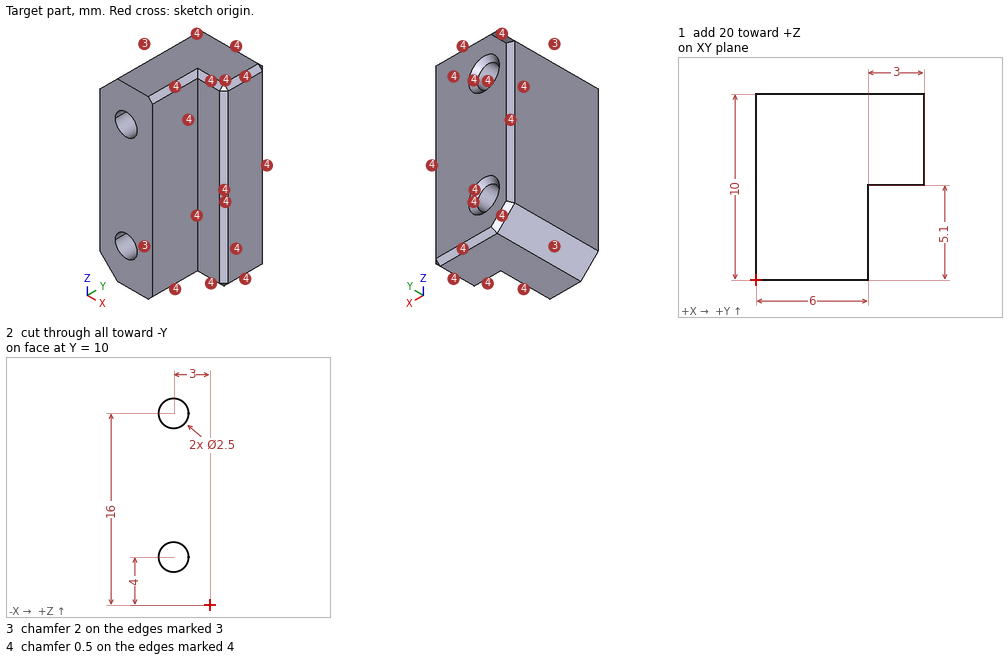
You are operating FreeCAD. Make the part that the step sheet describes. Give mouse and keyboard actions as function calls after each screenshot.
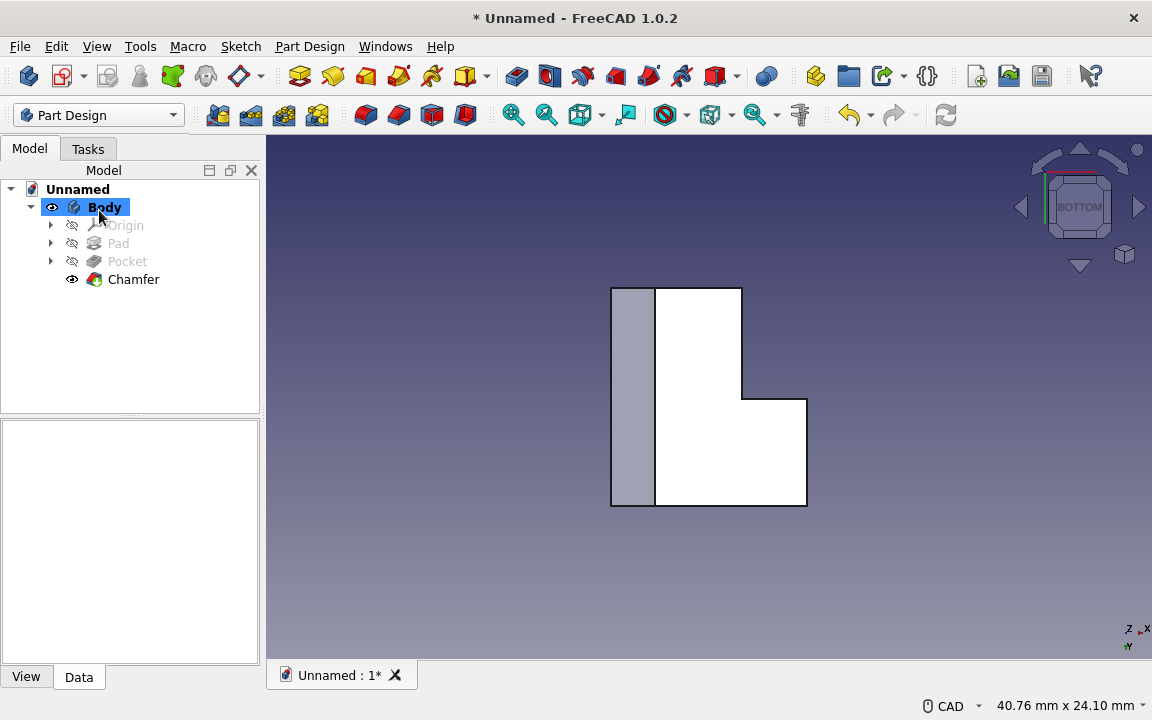
click(514, 116)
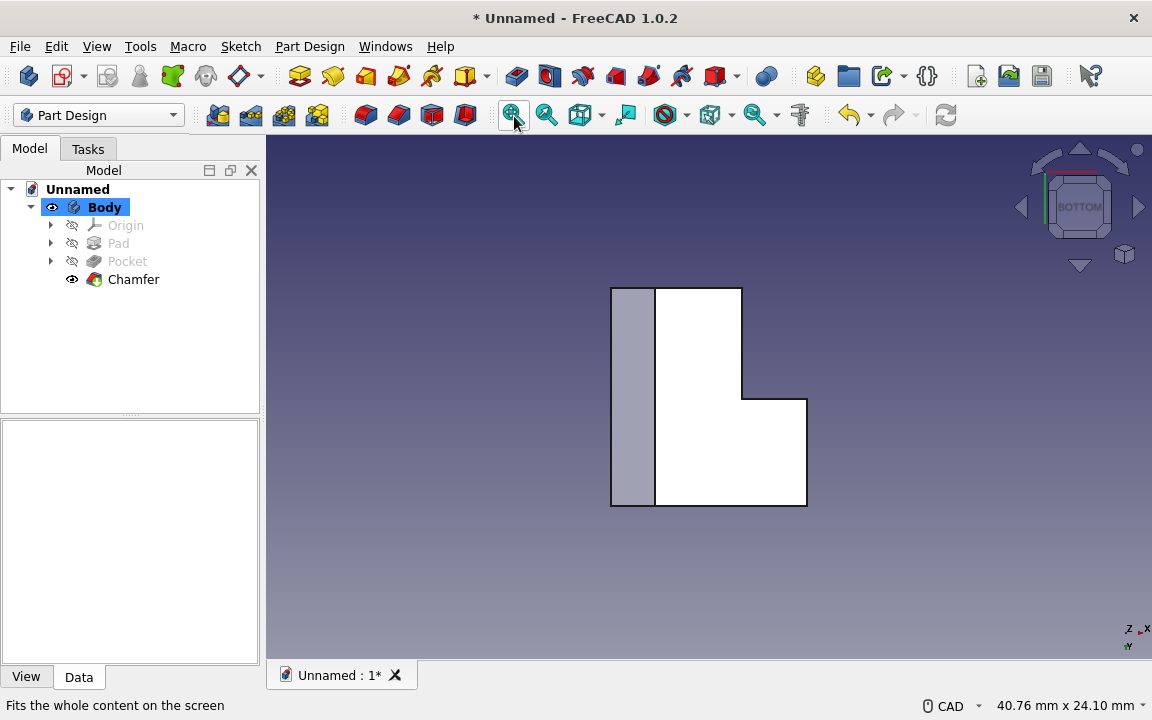
click(774, 398)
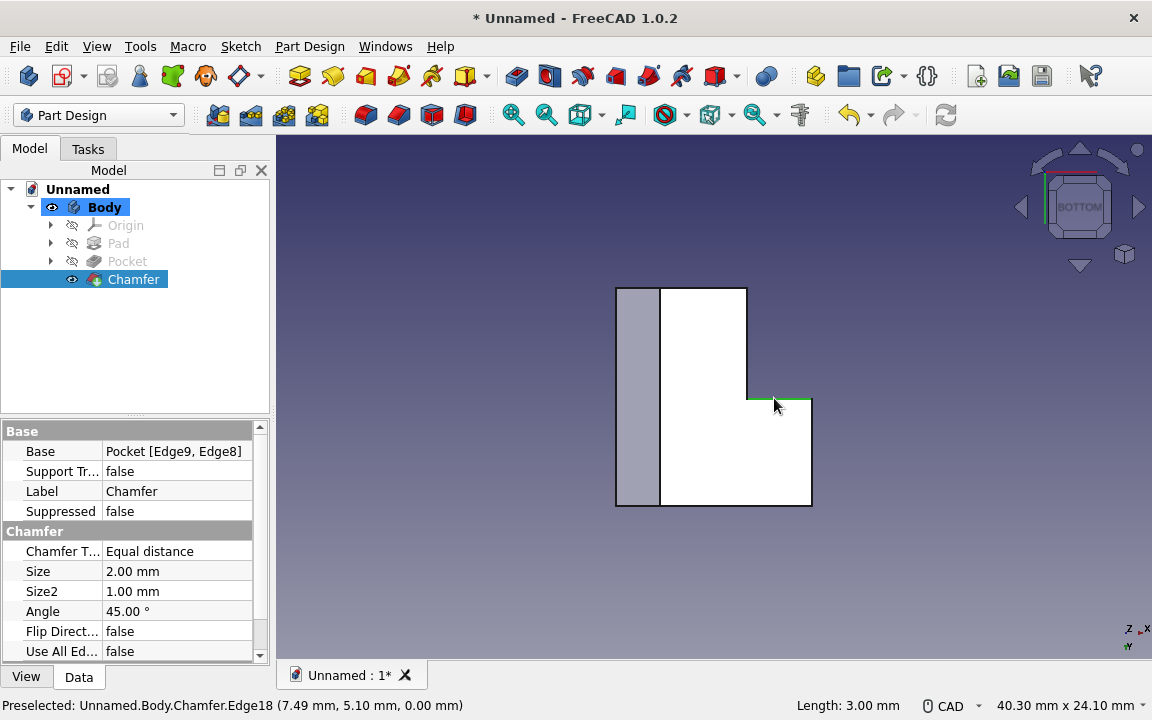
key(0)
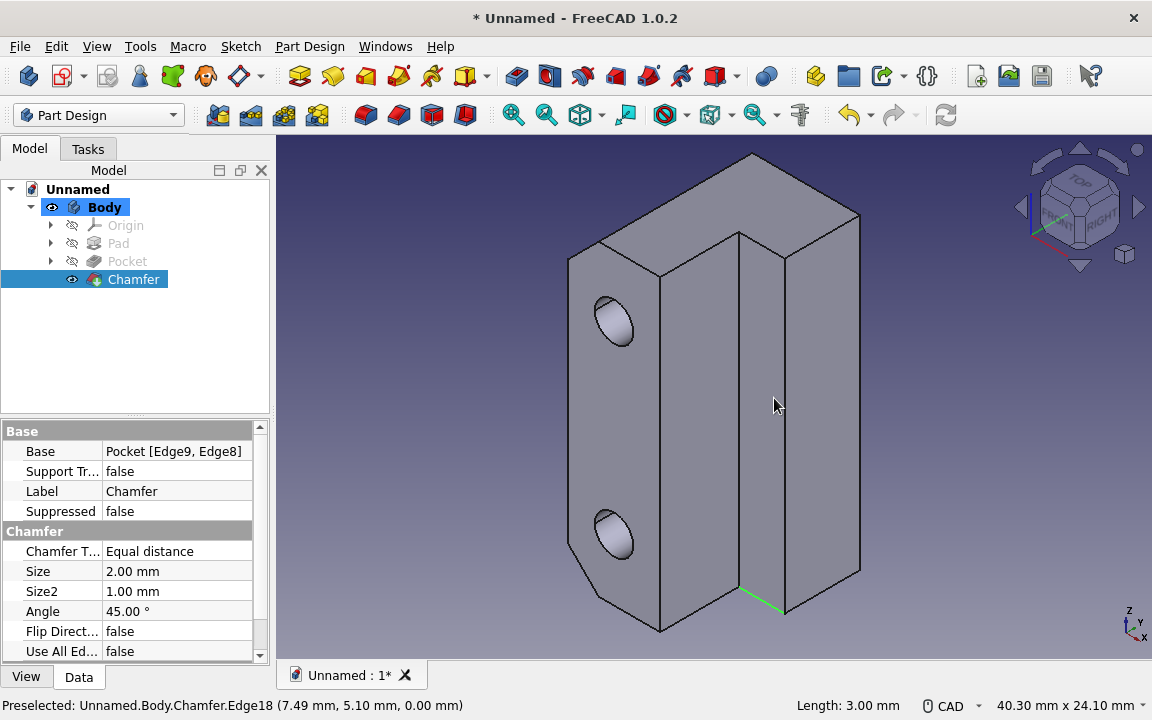
click(514, 116)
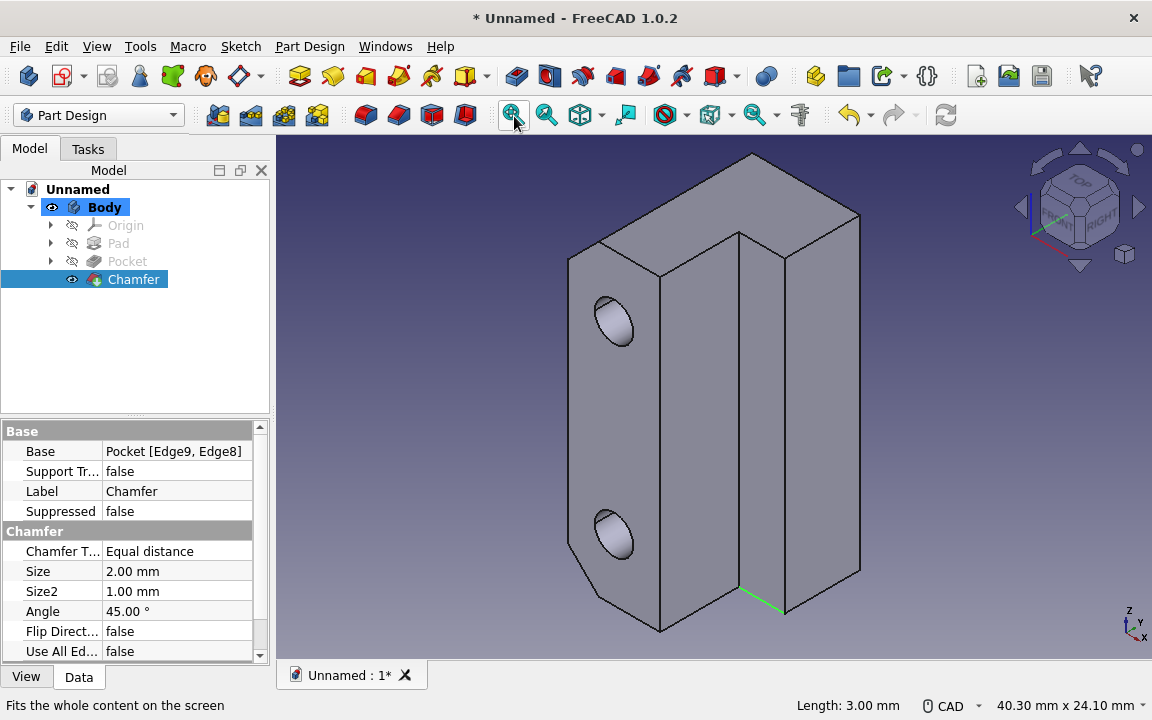
click(822, 312, ctrl)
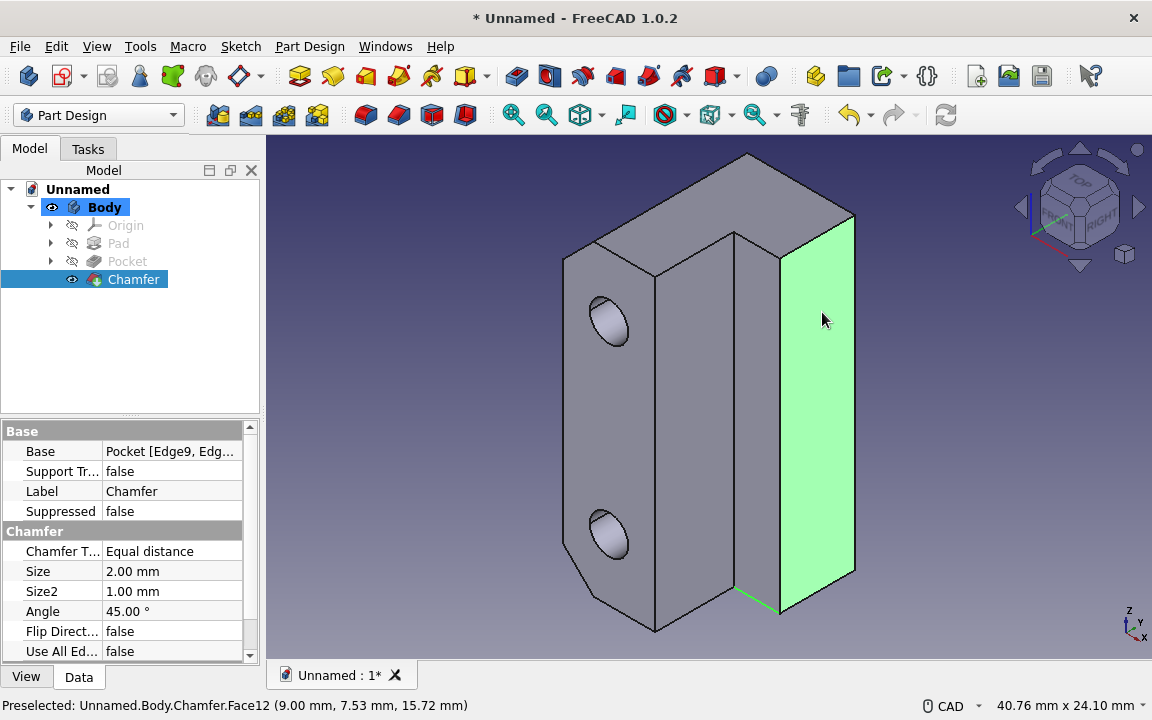
click(694, 254, ctrl)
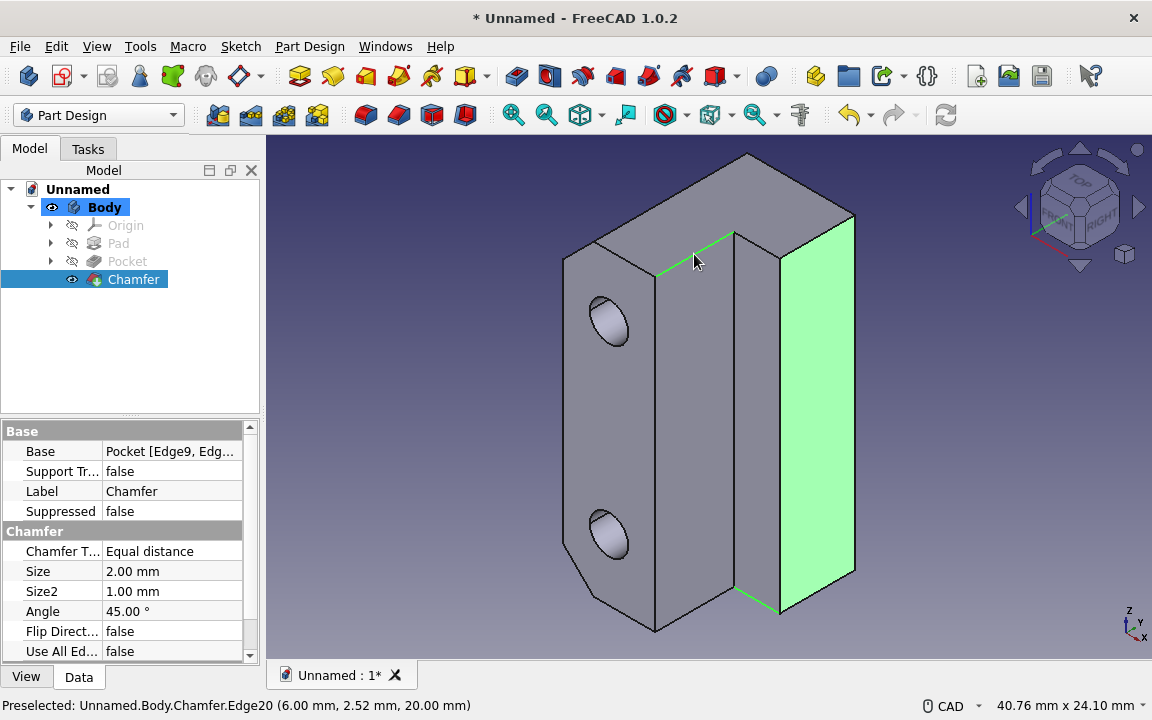
click(757, 244, ctrl)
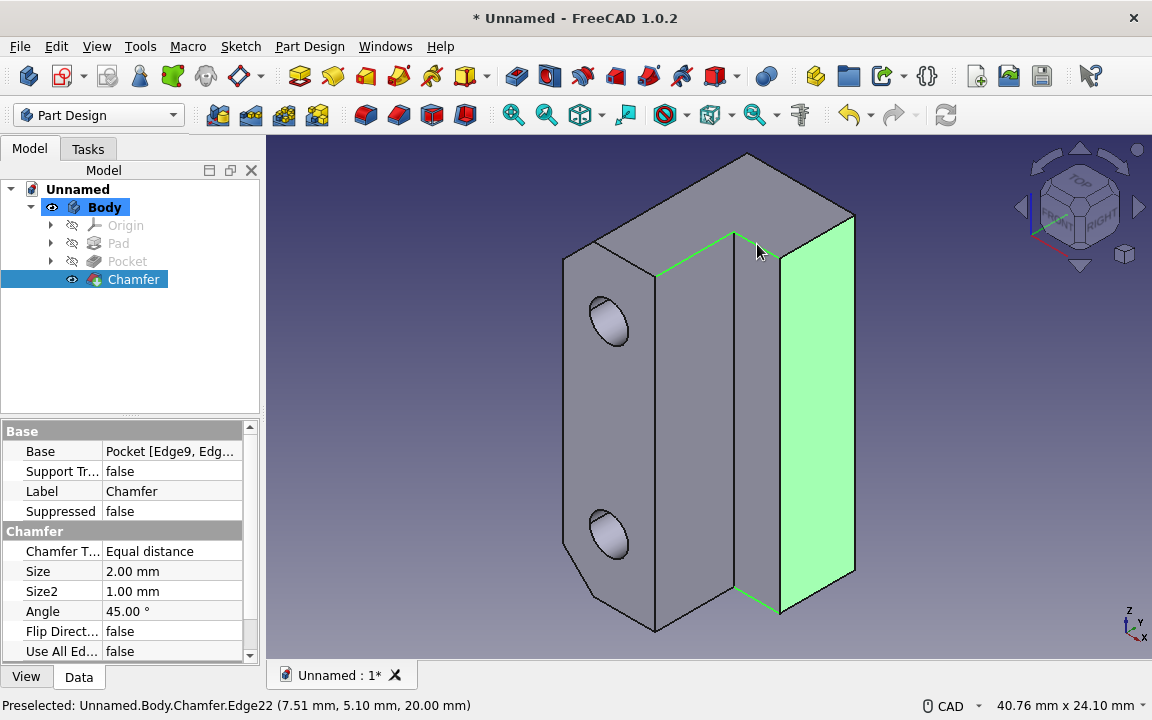
key(2)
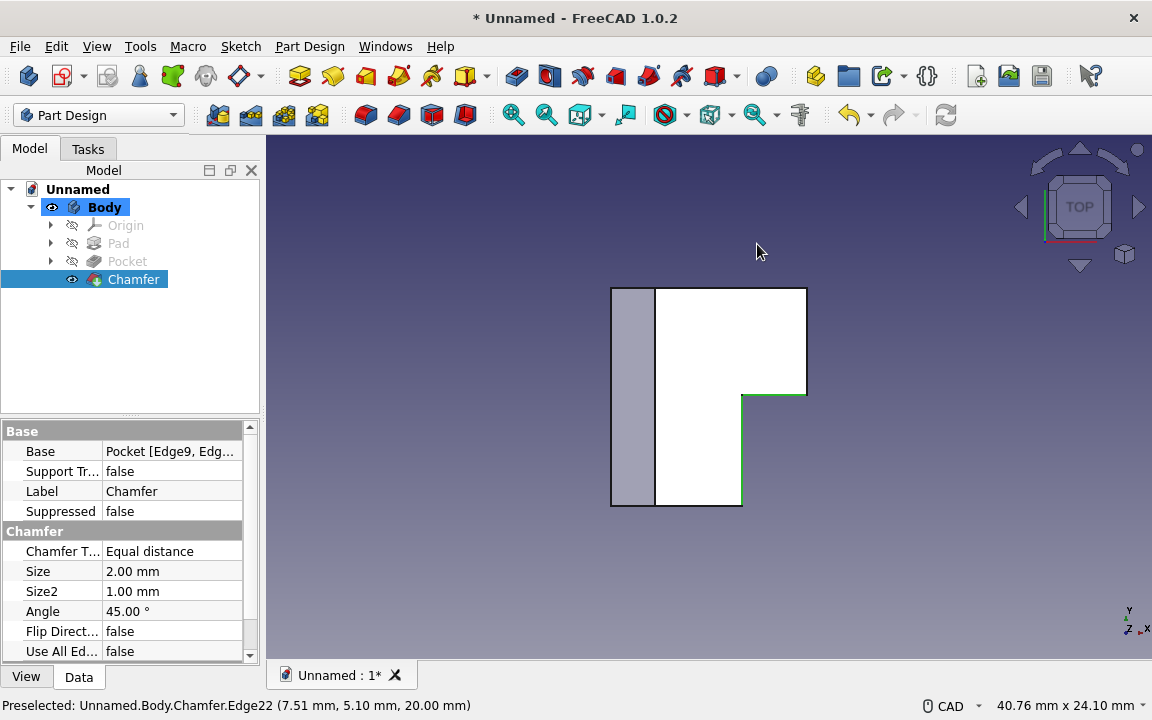
click(514, 116)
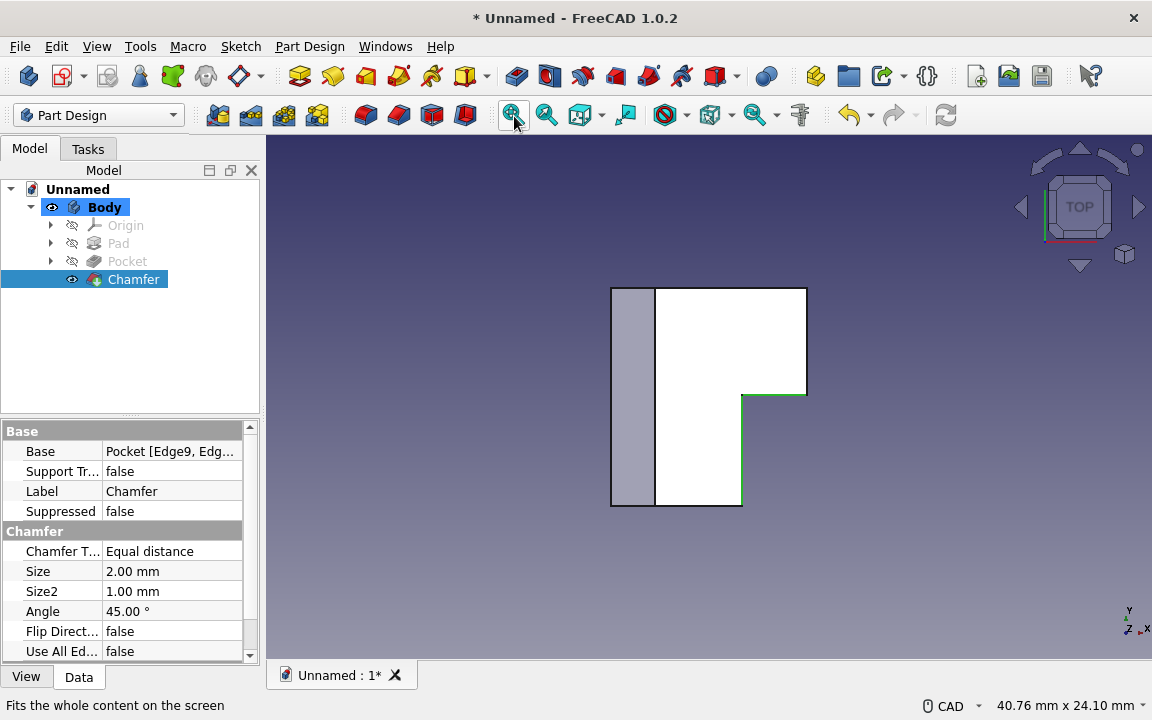
key(1)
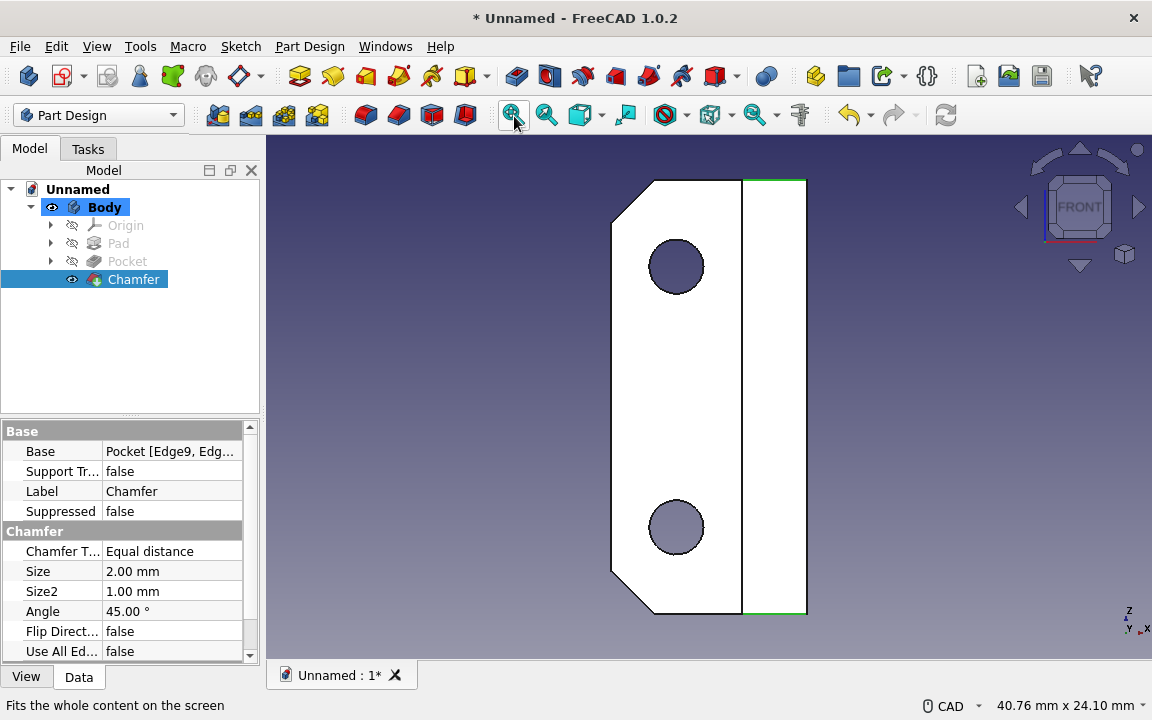
key(3)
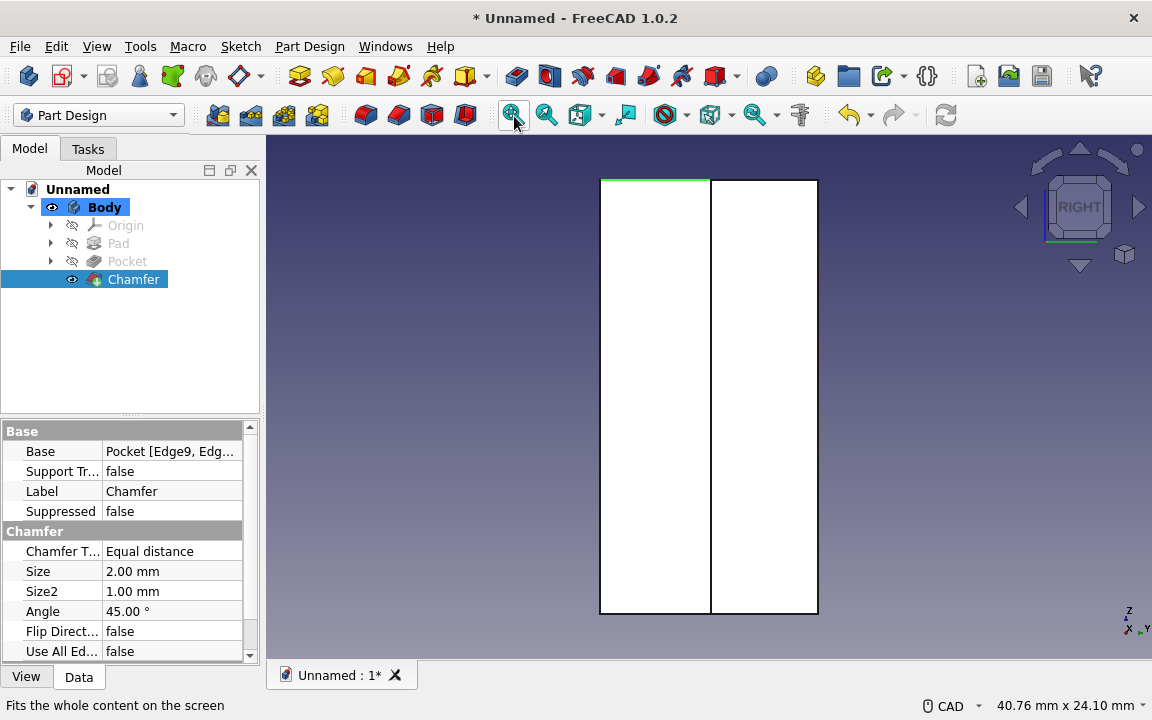
click(656, 613, ctrl)